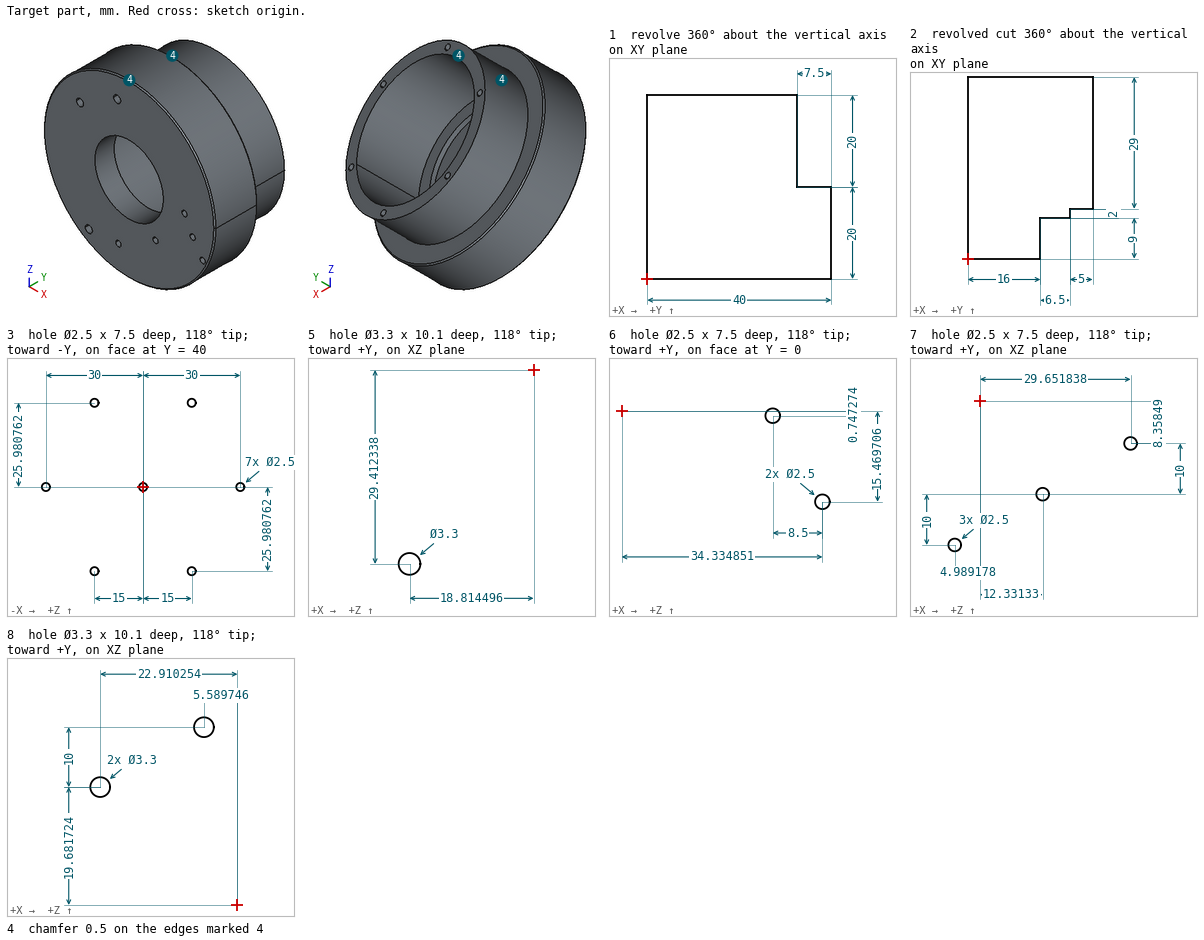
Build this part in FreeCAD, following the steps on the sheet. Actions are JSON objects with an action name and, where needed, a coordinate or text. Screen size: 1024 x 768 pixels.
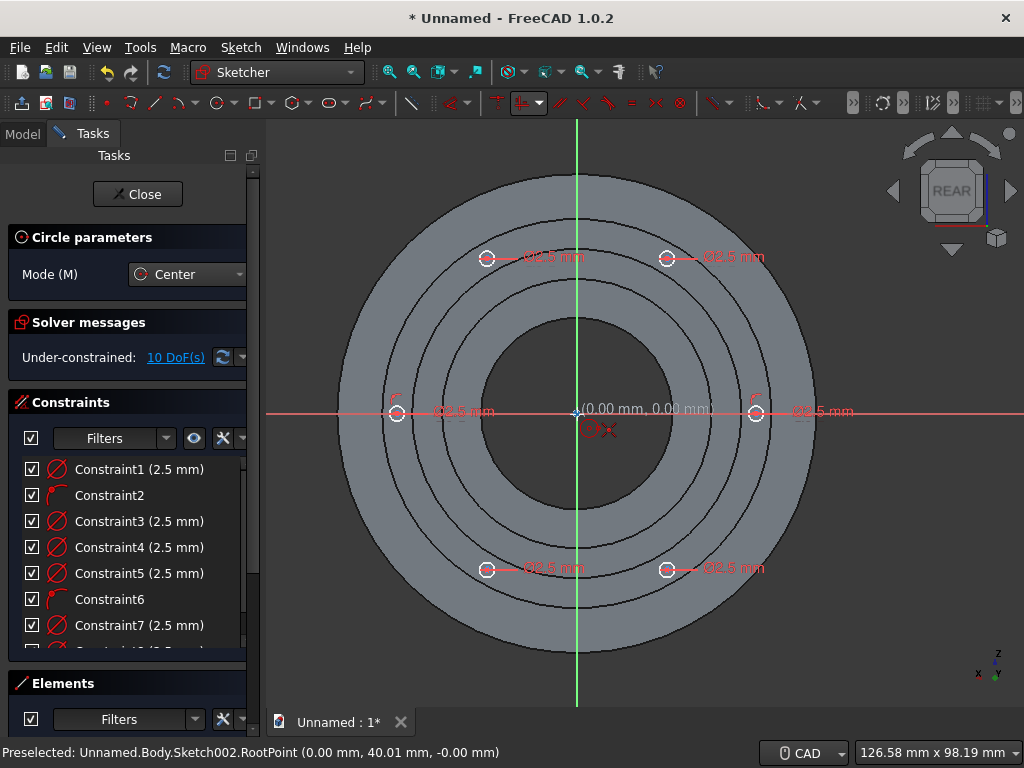
{"action": "left_click", "coordinate": [577, 414]}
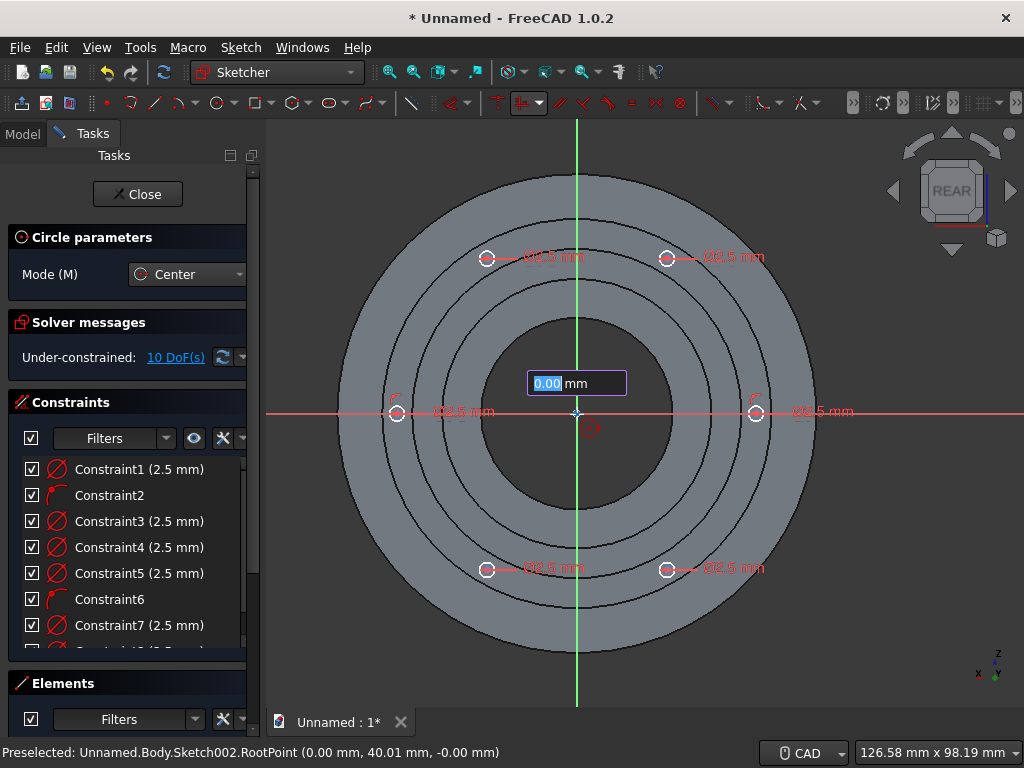
{"action": "scroll", "coordinate": [582, 408], "scroll_direction": "up", "scroll_amount": 6}
{"action": "mouse_move", "coordinate": [581, 408]}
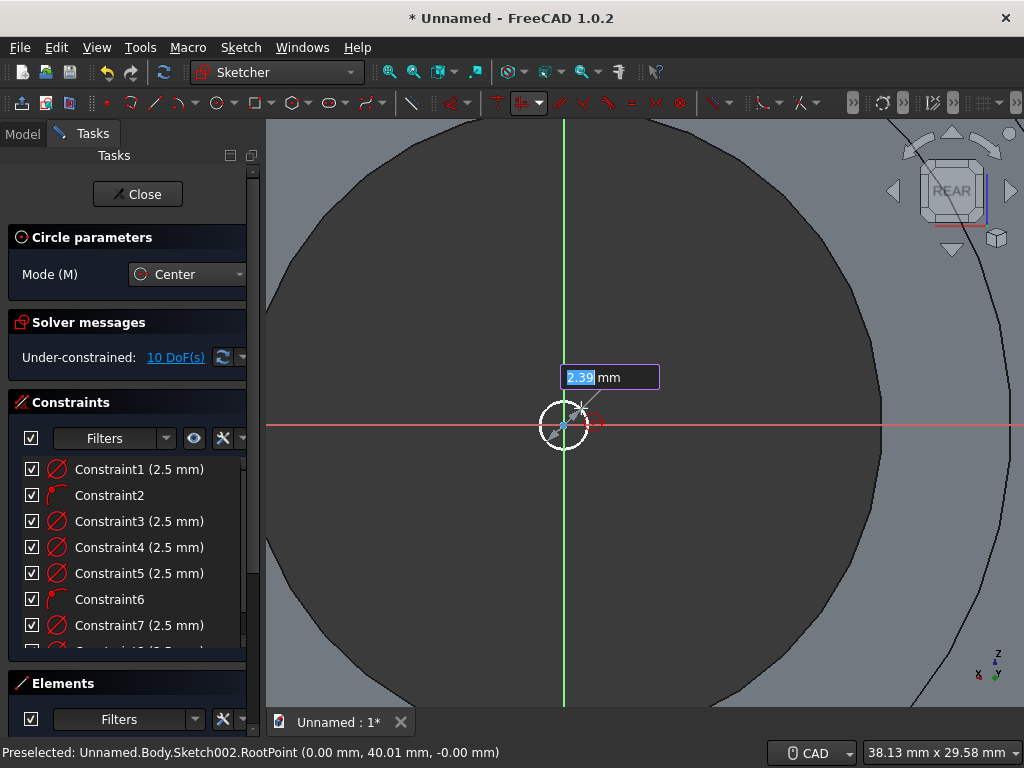
{"action": "type", "text": "2.5"}
{"action": "key", "text": "Return"}
{"action": "key", "text": "Escape"}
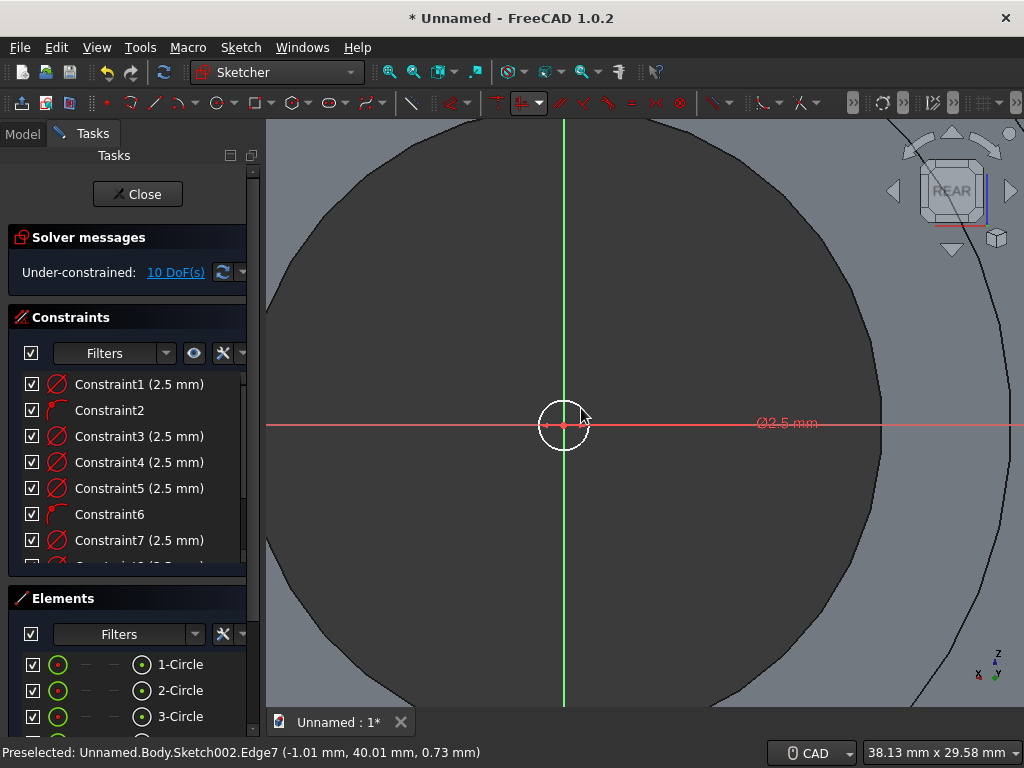
{"action": "scroll", "coordinate": [582, 408], "scroll_direction": "down", "scroll_amount": 6}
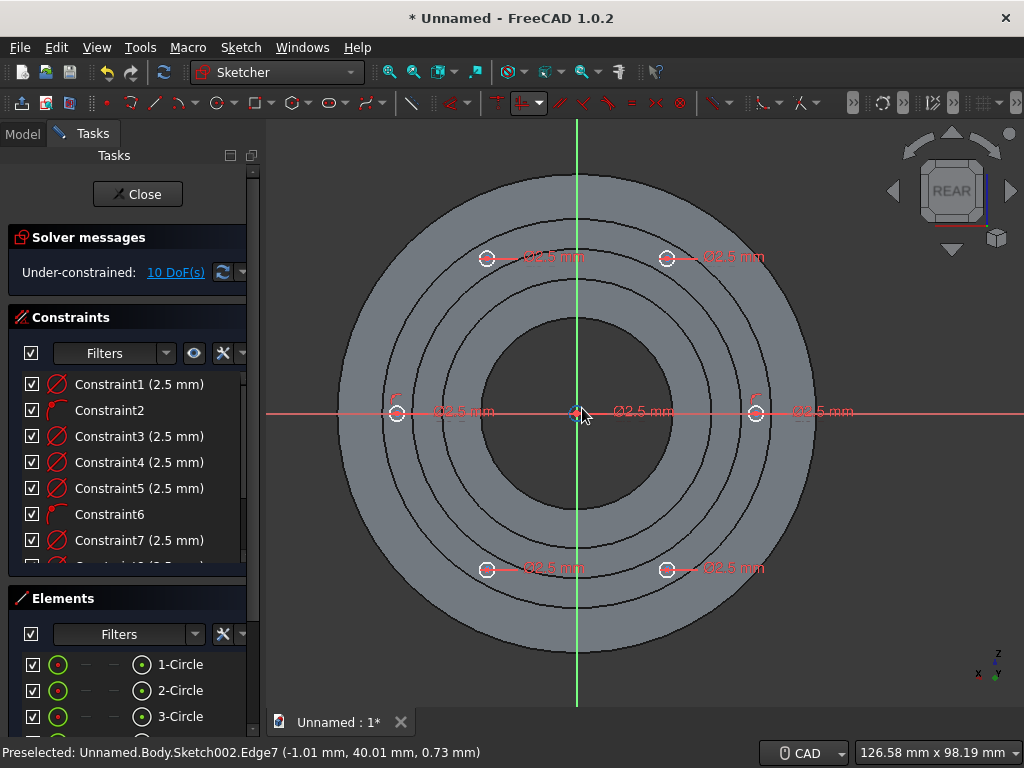
{"action": "left_click", "coordinate": [667, 570]}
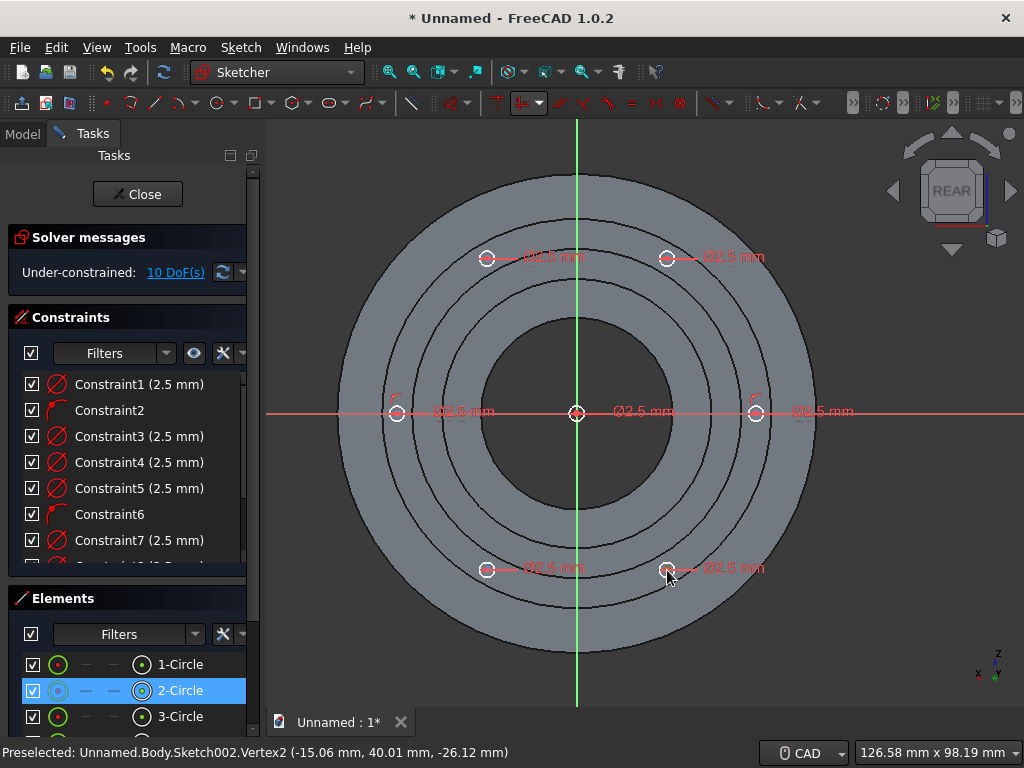
{"action": "left_click", "coordinate": [487, 570]}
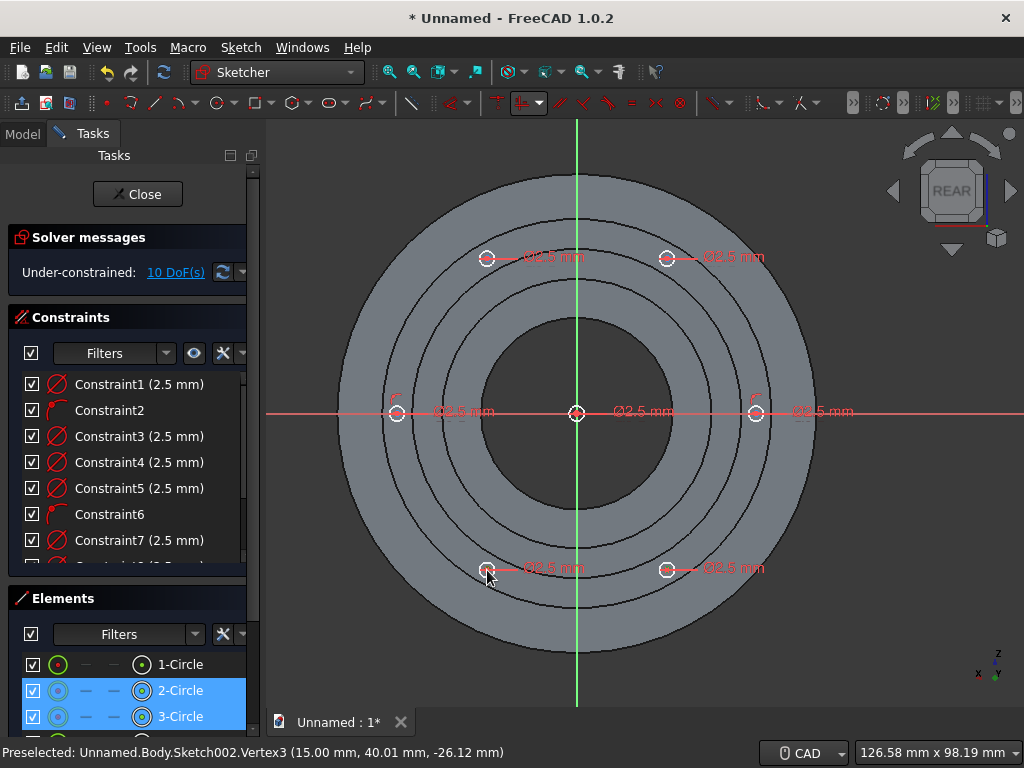
{"action": "key", "text": "h"}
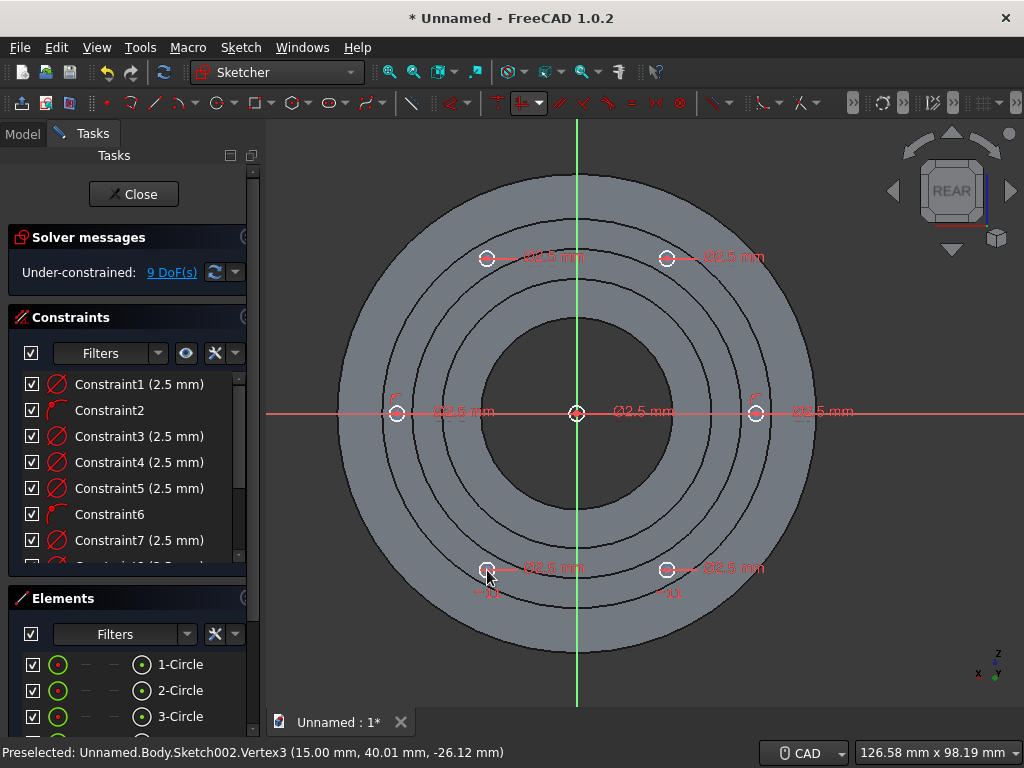
{"action": "left_click", "coordinate": [487, 570]}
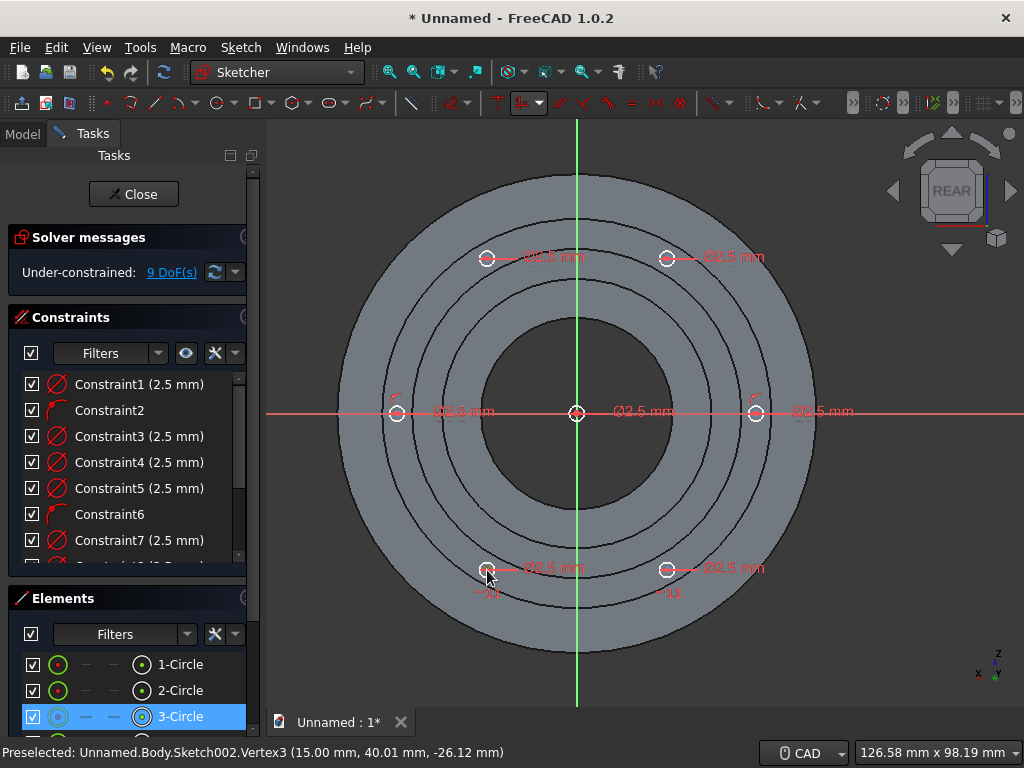
{"action": "left_click", "coordinate": [487, 259]}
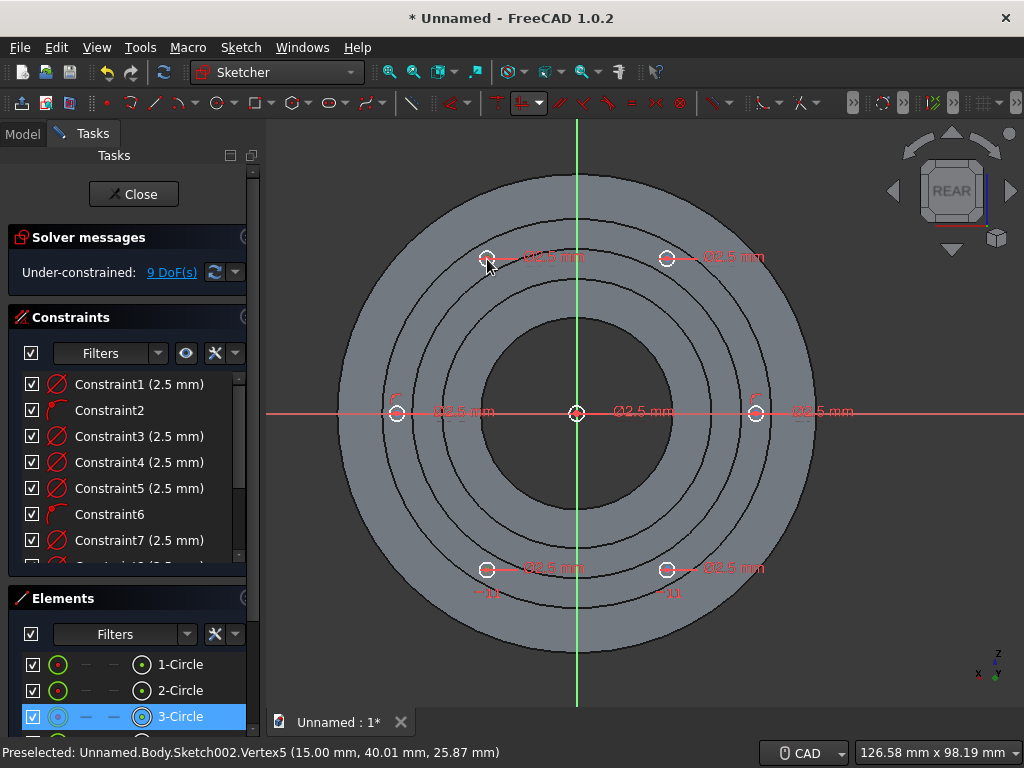
{"action": "key", "text": "v"}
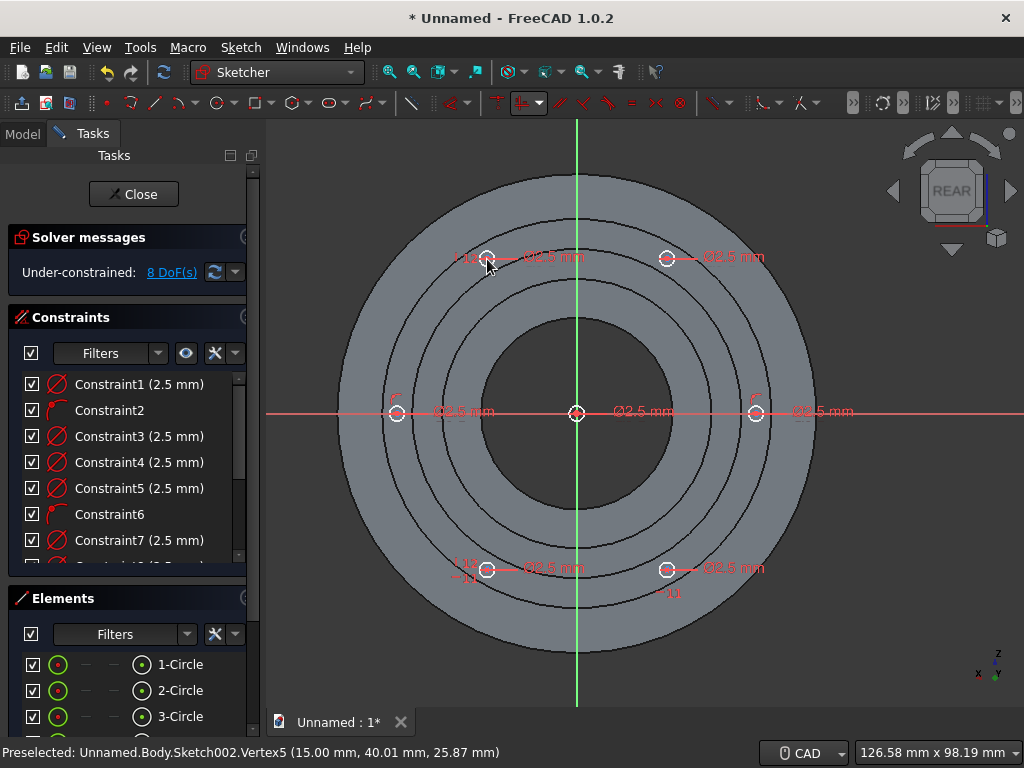
{"action": "left_click", "coordinate": [667, 570]}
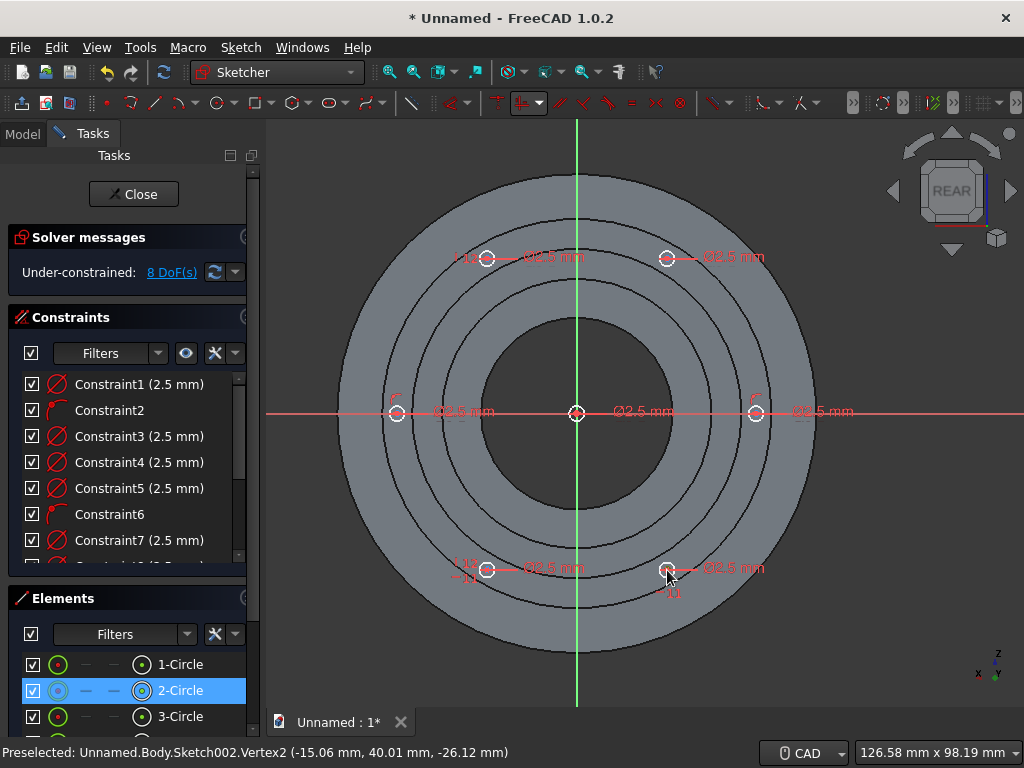
{"action": "left_click", "coordinate": [667, 259]}